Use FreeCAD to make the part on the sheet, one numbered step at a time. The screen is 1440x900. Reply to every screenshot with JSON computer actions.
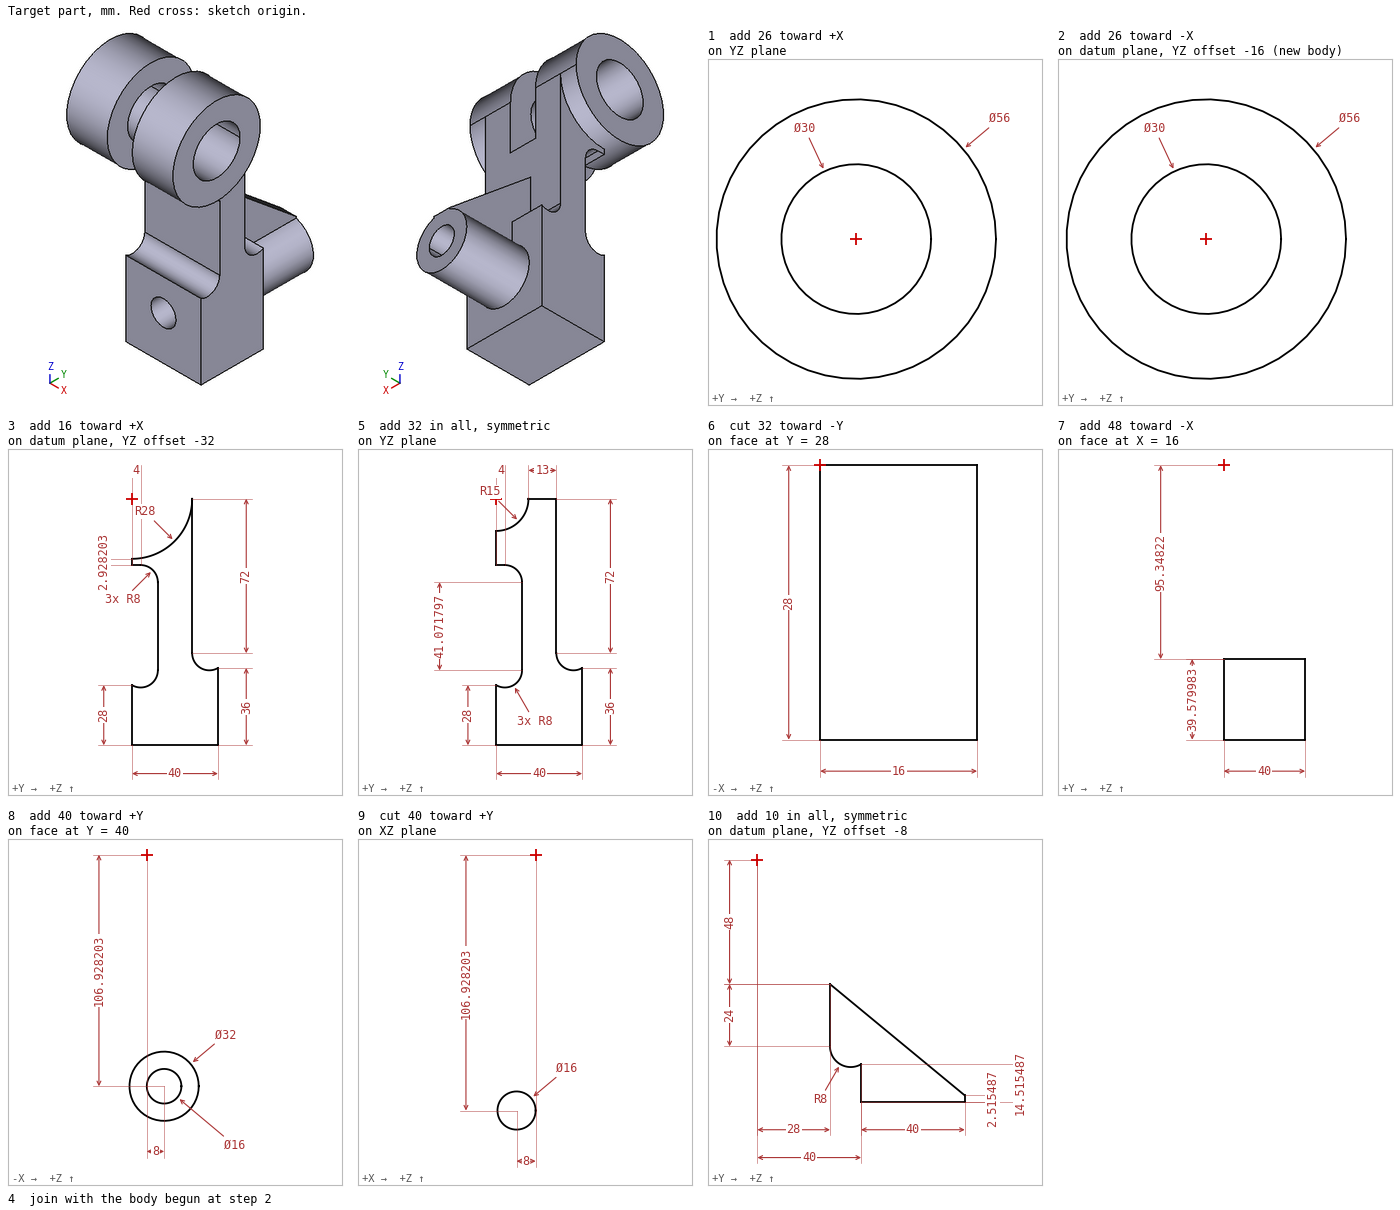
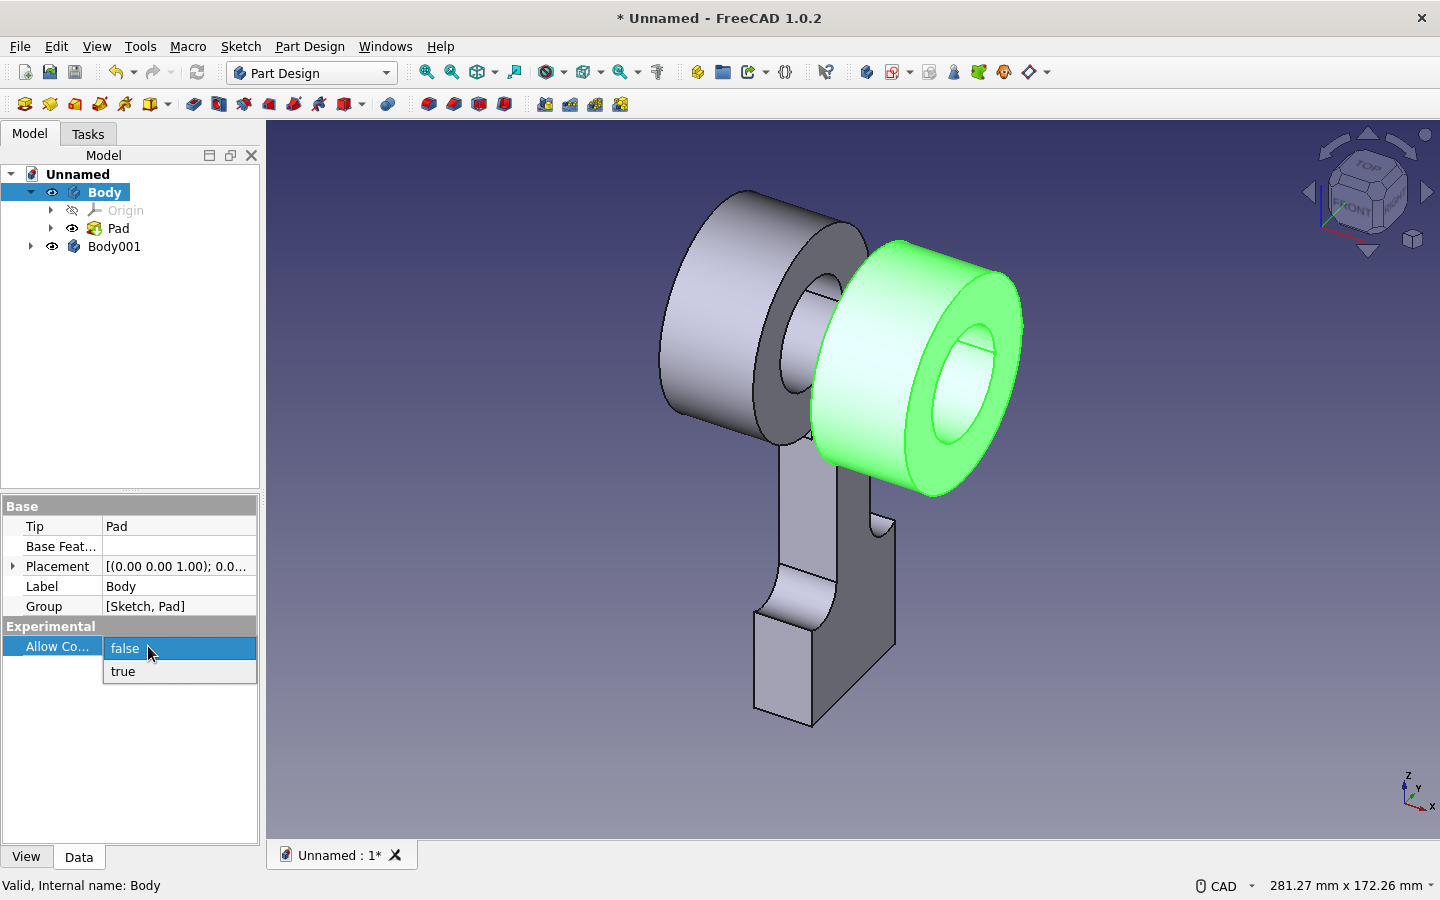
{"action": "left_click", "coordinate": [178, 672]}
{"action": "key", "text": "Return"}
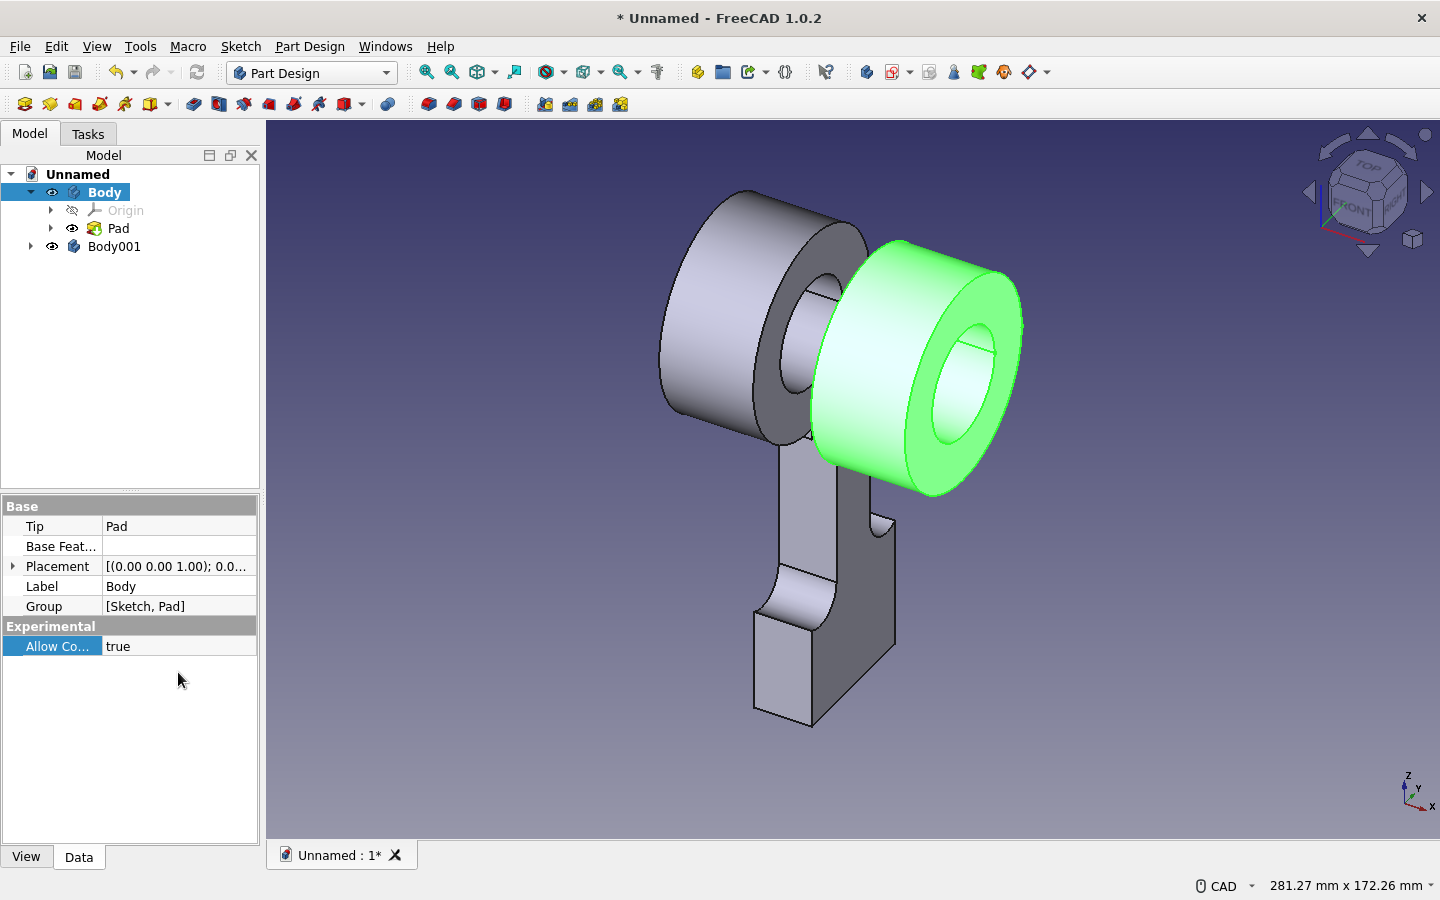
{"action": "left_click", "coordinate": [97, 246]}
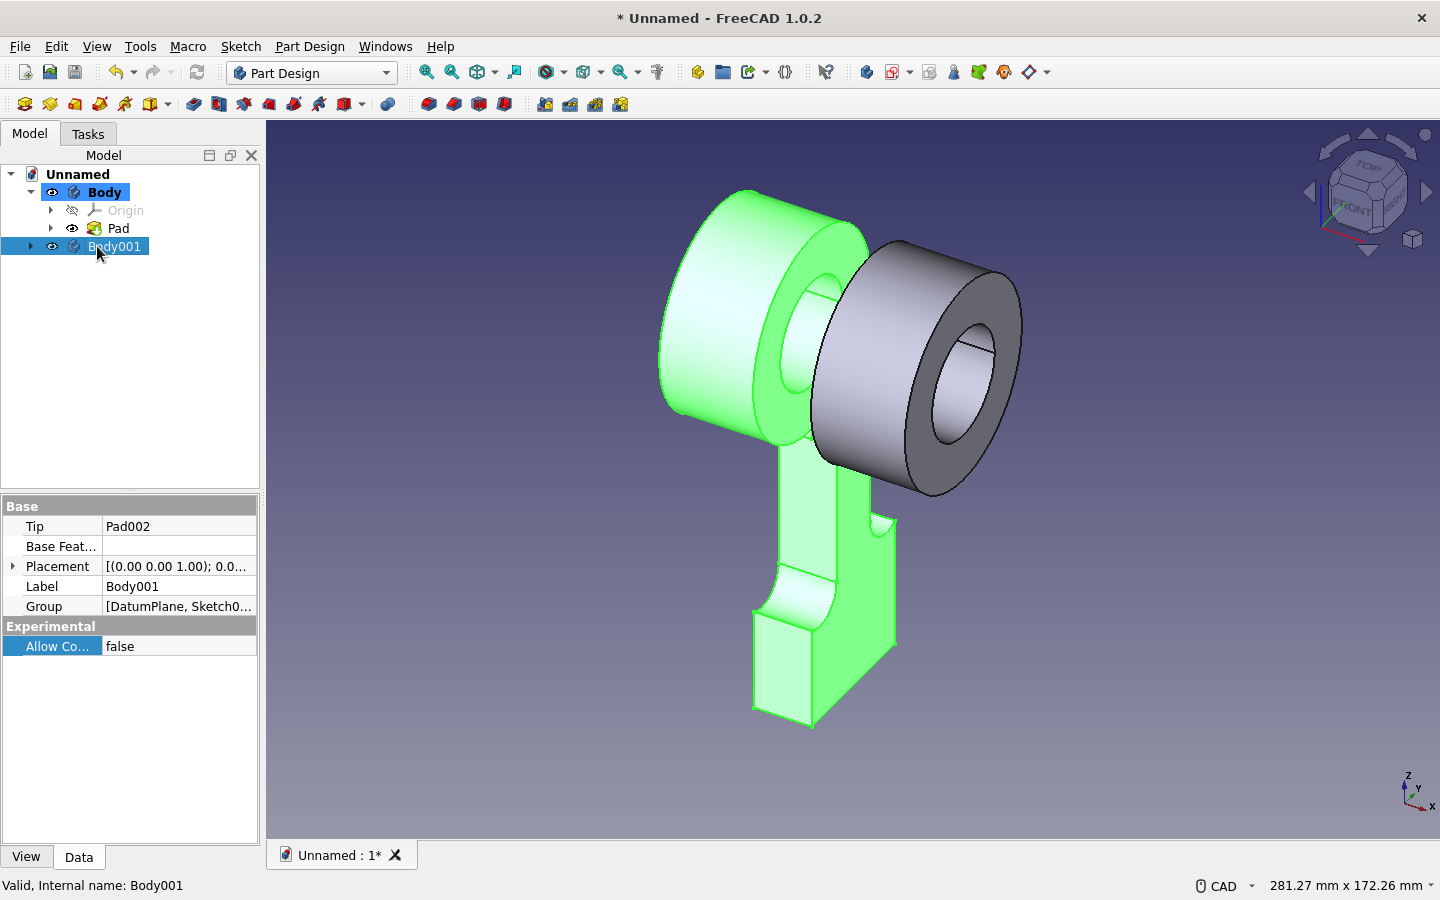
{"action": "left_click", "coordinate": [388, 104]}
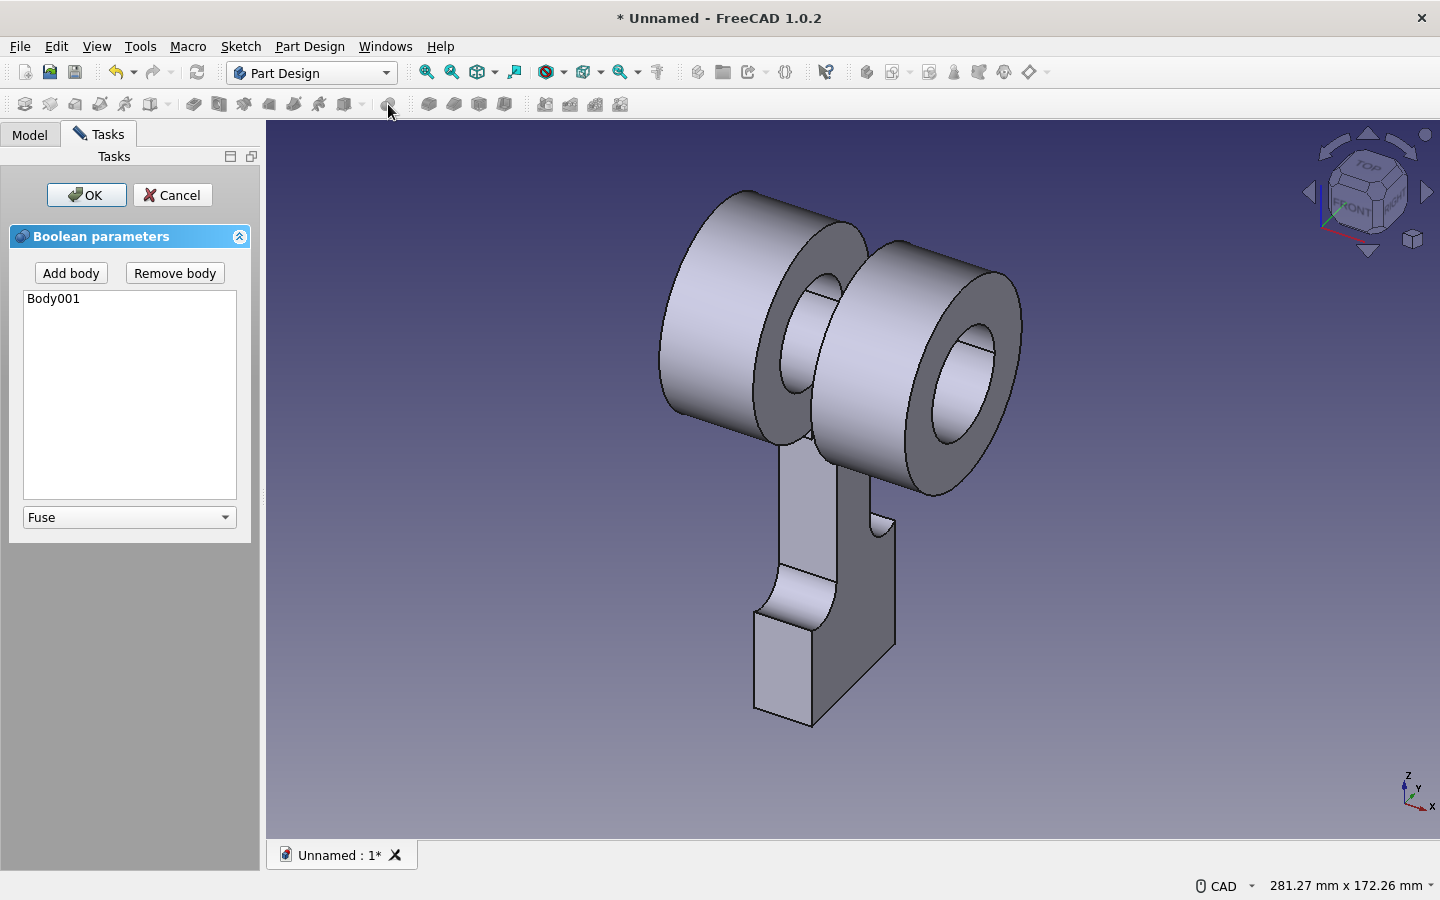
{"action": "left_click", "coordinate": [87, 195]}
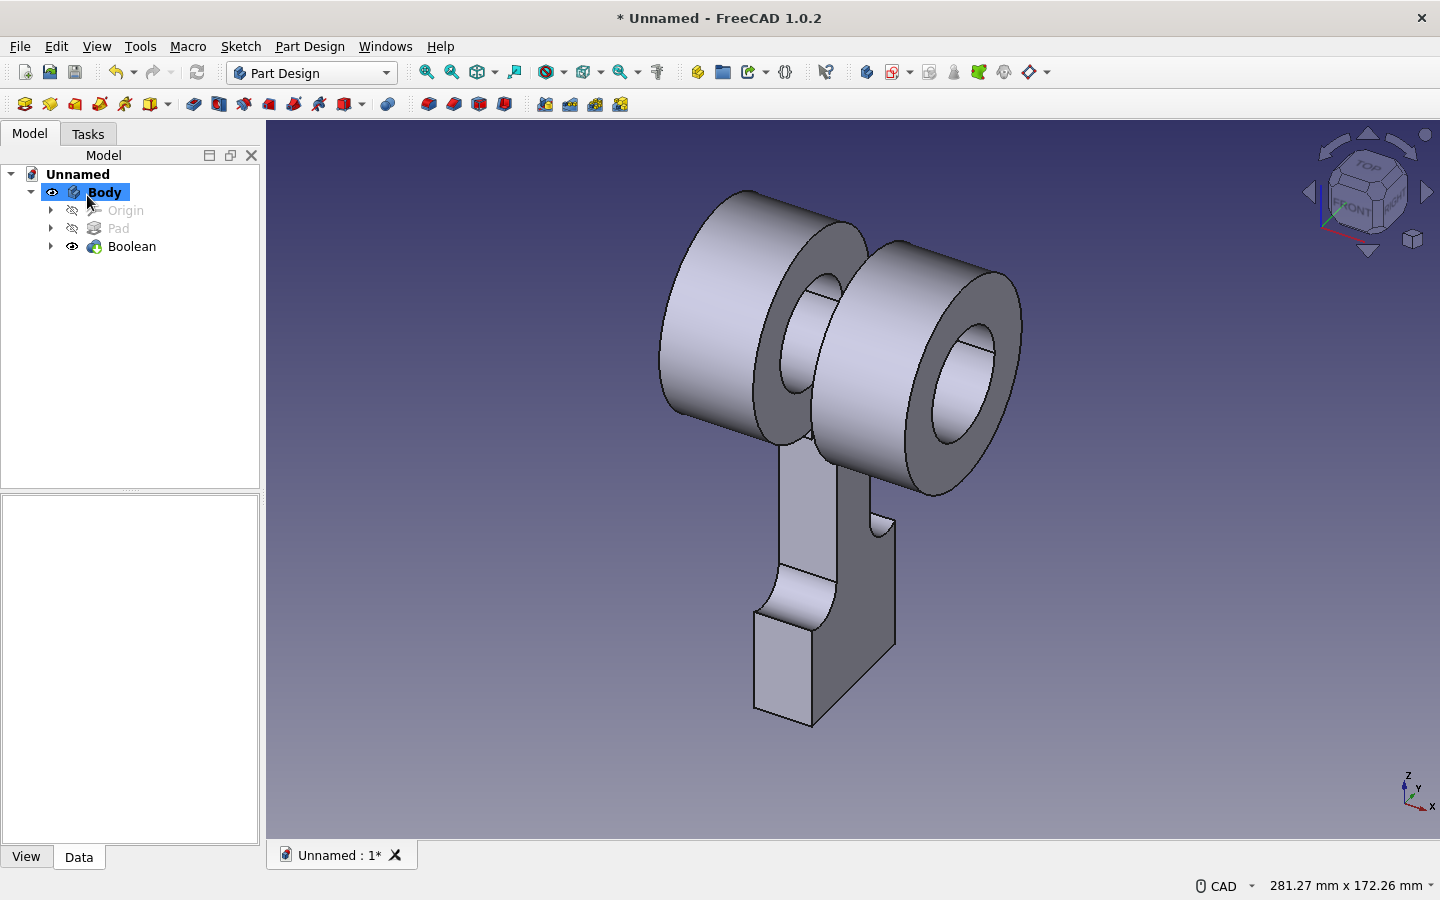
{"action": "left_click", "coordinate": [892, 72]}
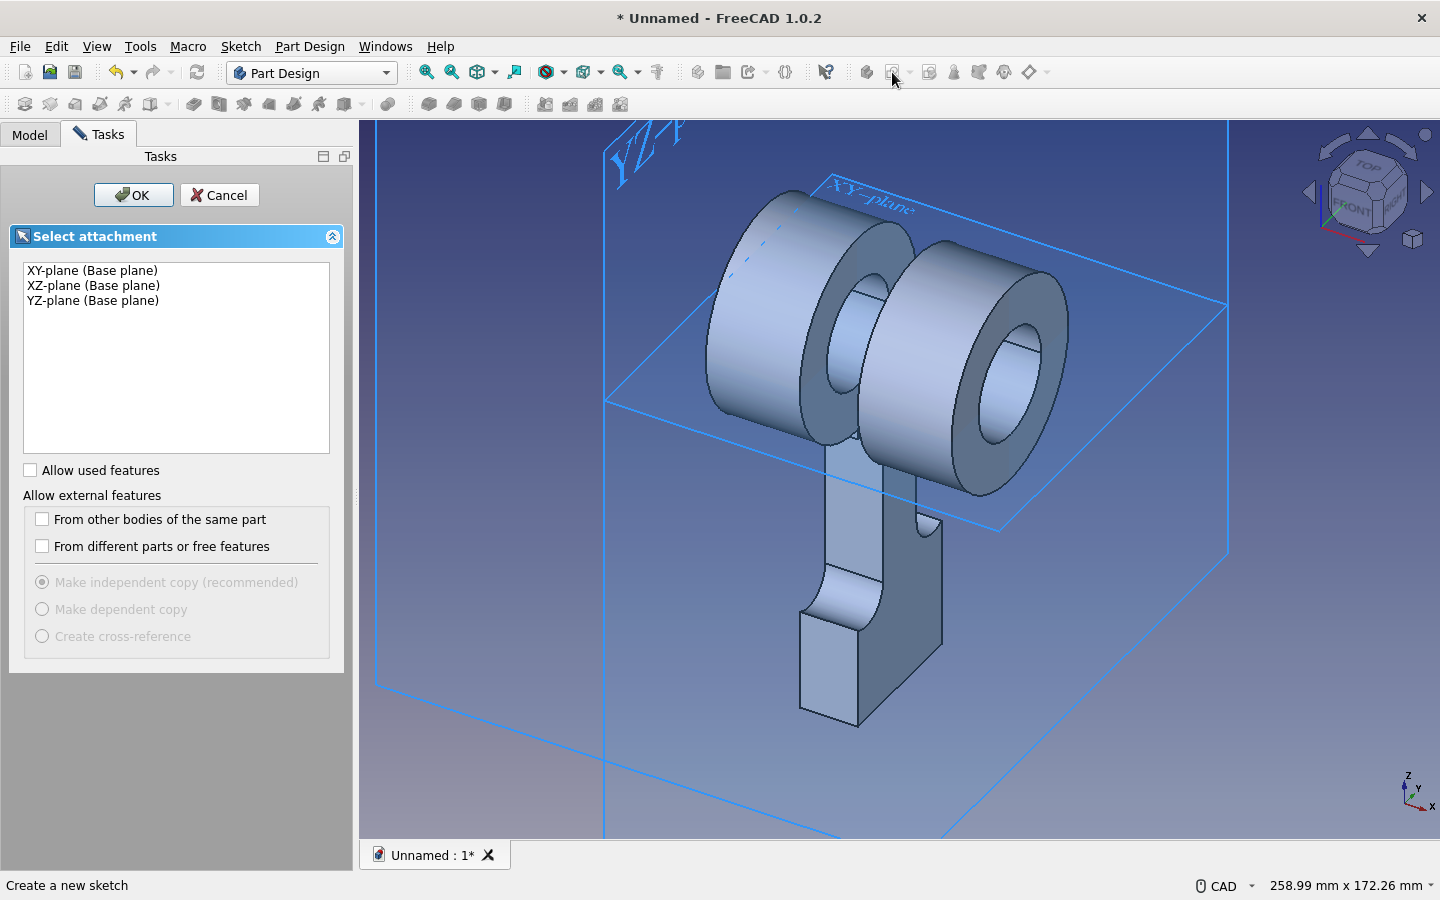
{"action": "left_click", "coordinate": [84, 300]}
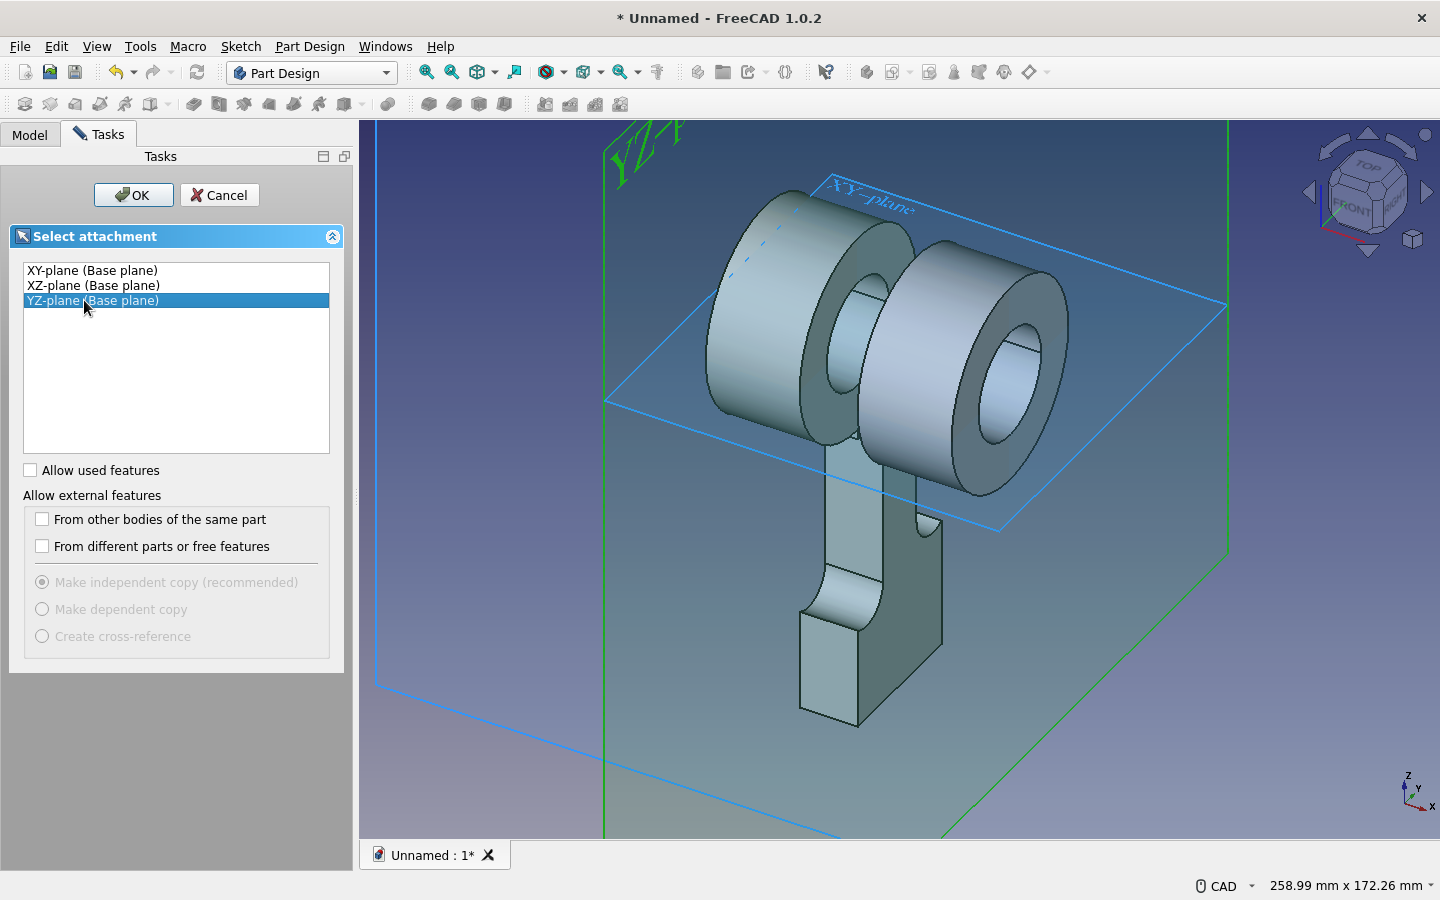
{"action": "left_click", "coordinate": [134, 195]}